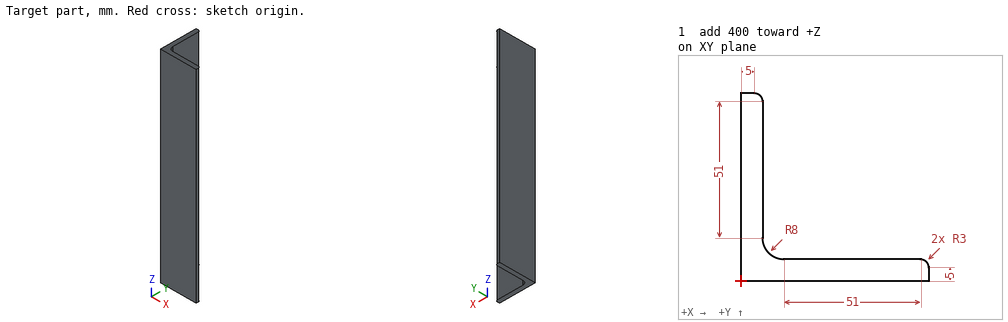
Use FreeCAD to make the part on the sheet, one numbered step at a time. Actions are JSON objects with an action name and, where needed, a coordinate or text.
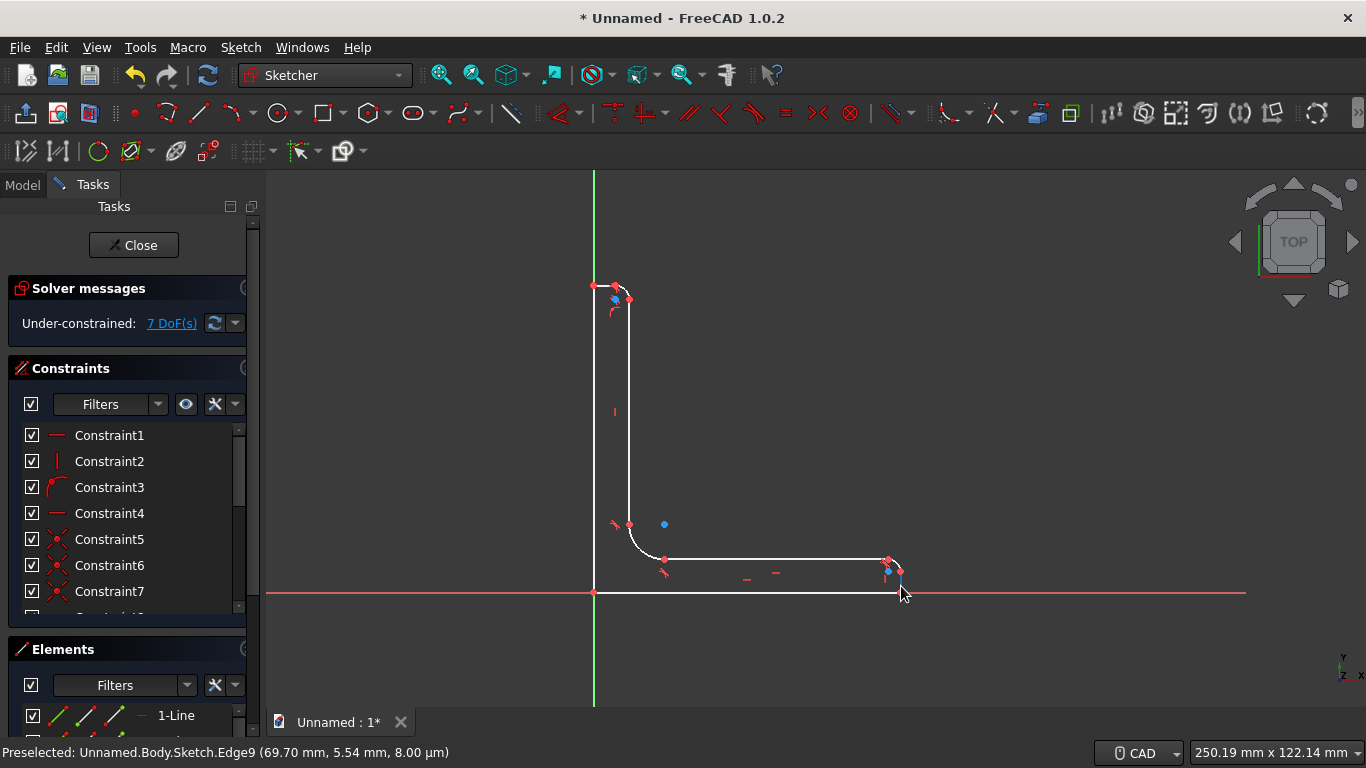
{"action": "scroll", "coordinate": [628, 293], "scroll_direction": "up", "scroll_amount": 4}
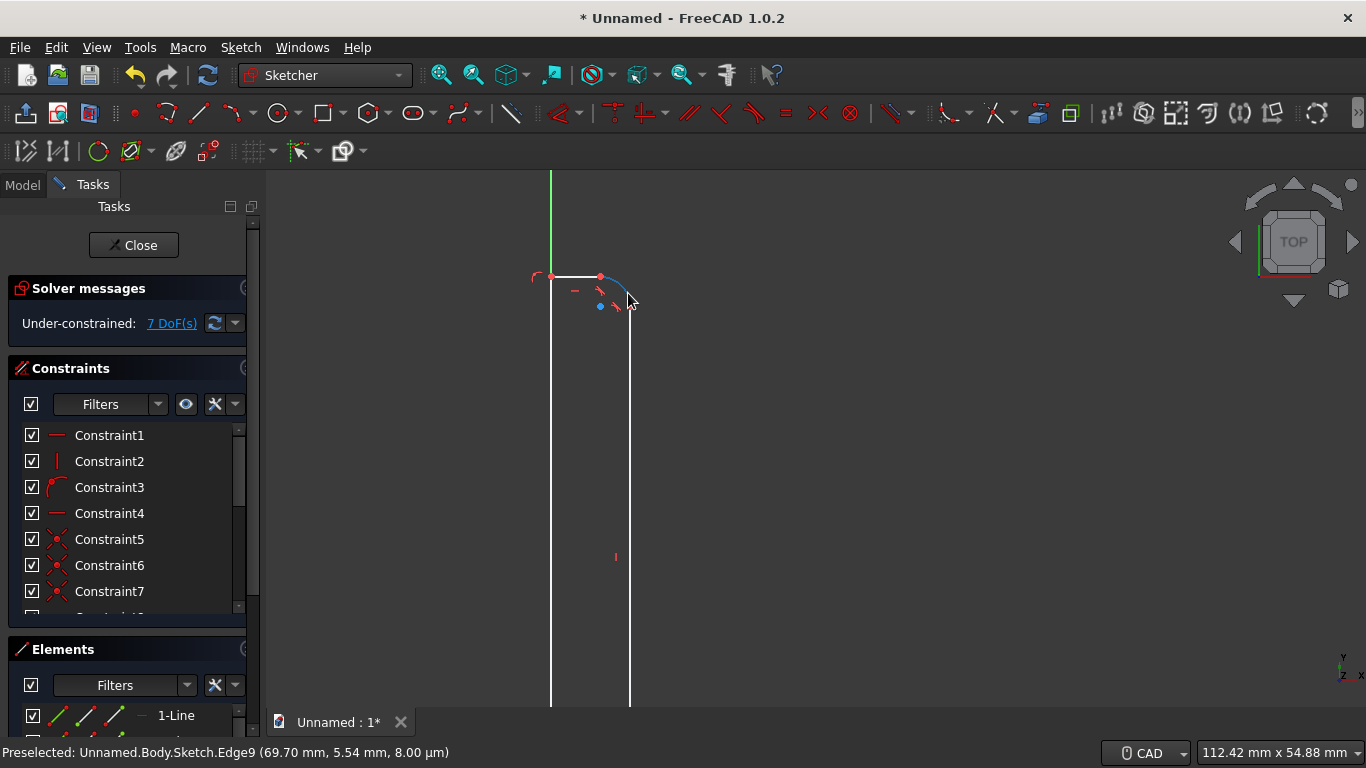
{"action": "left_click", "coordinate": [627, 293]}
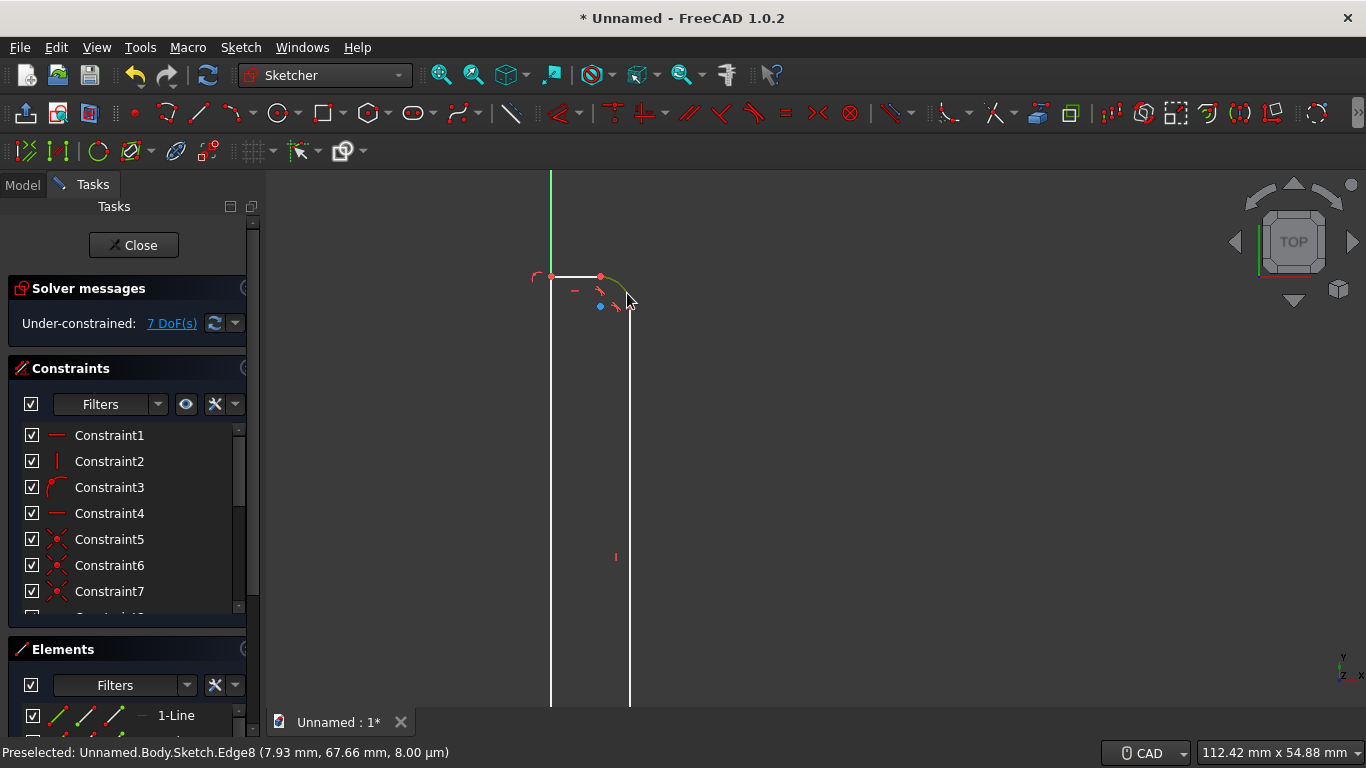
{"action": "scroll", "coordinate": [628, 293], "scroll_direction": "down", "scroll_amount": 4}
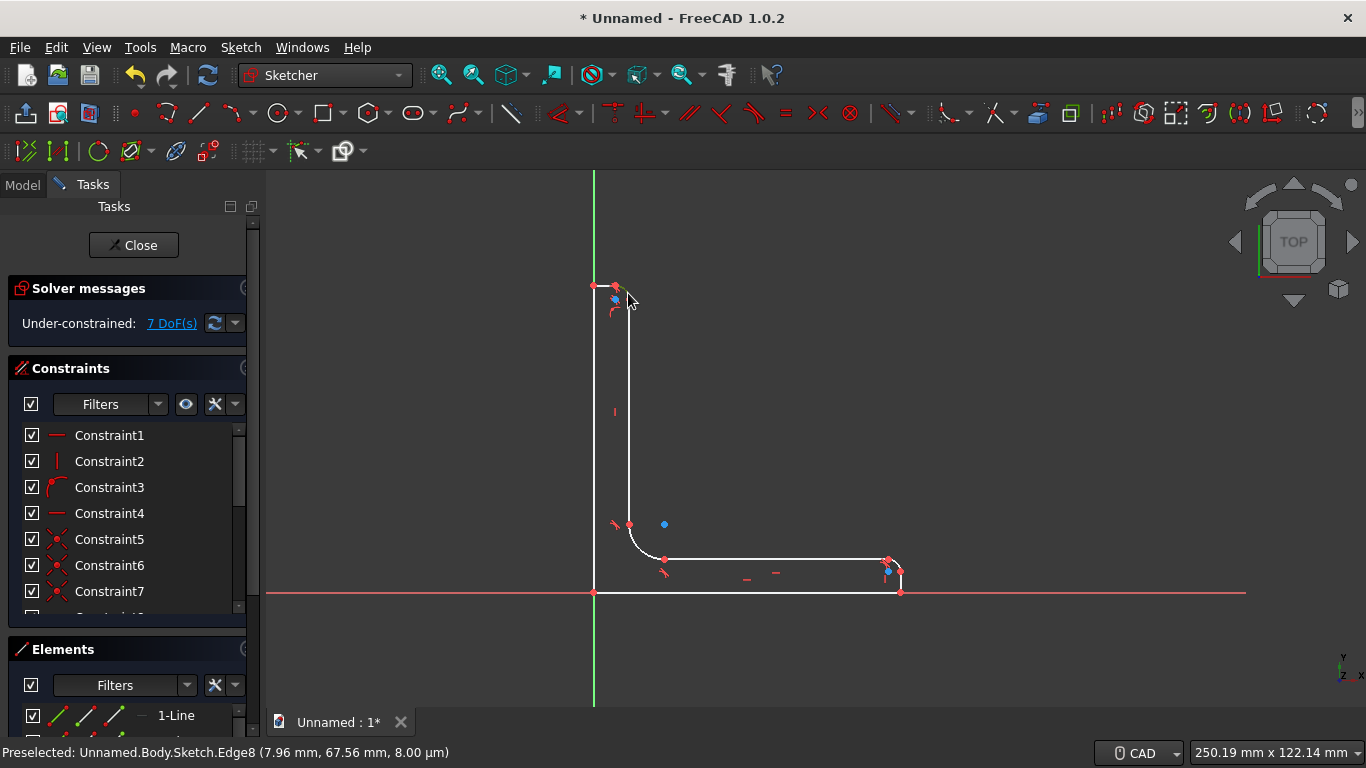
{"action": "scroll", "coordinate": [899, 566], "scroll_direction": "up", "scroll_amount": 5}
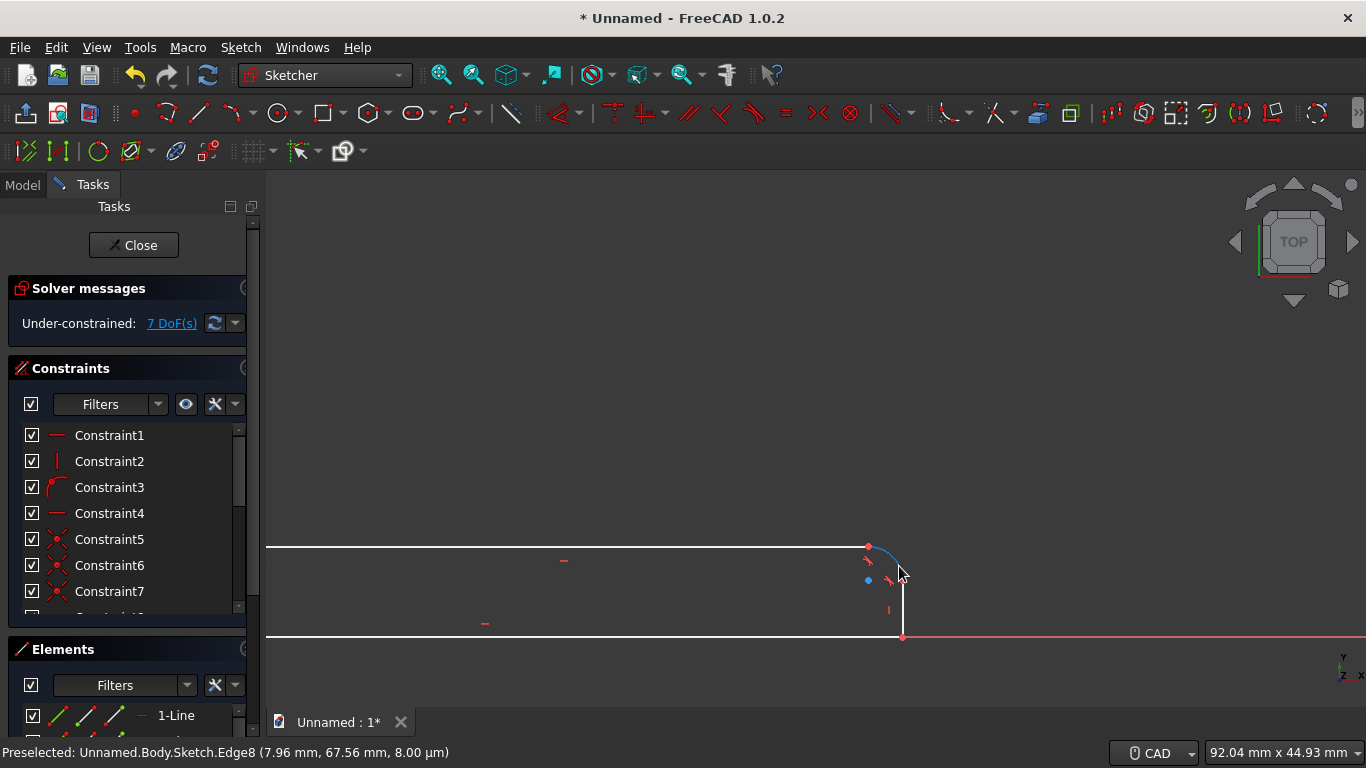
{"action": "left_click", "coordinate": [899, 565]}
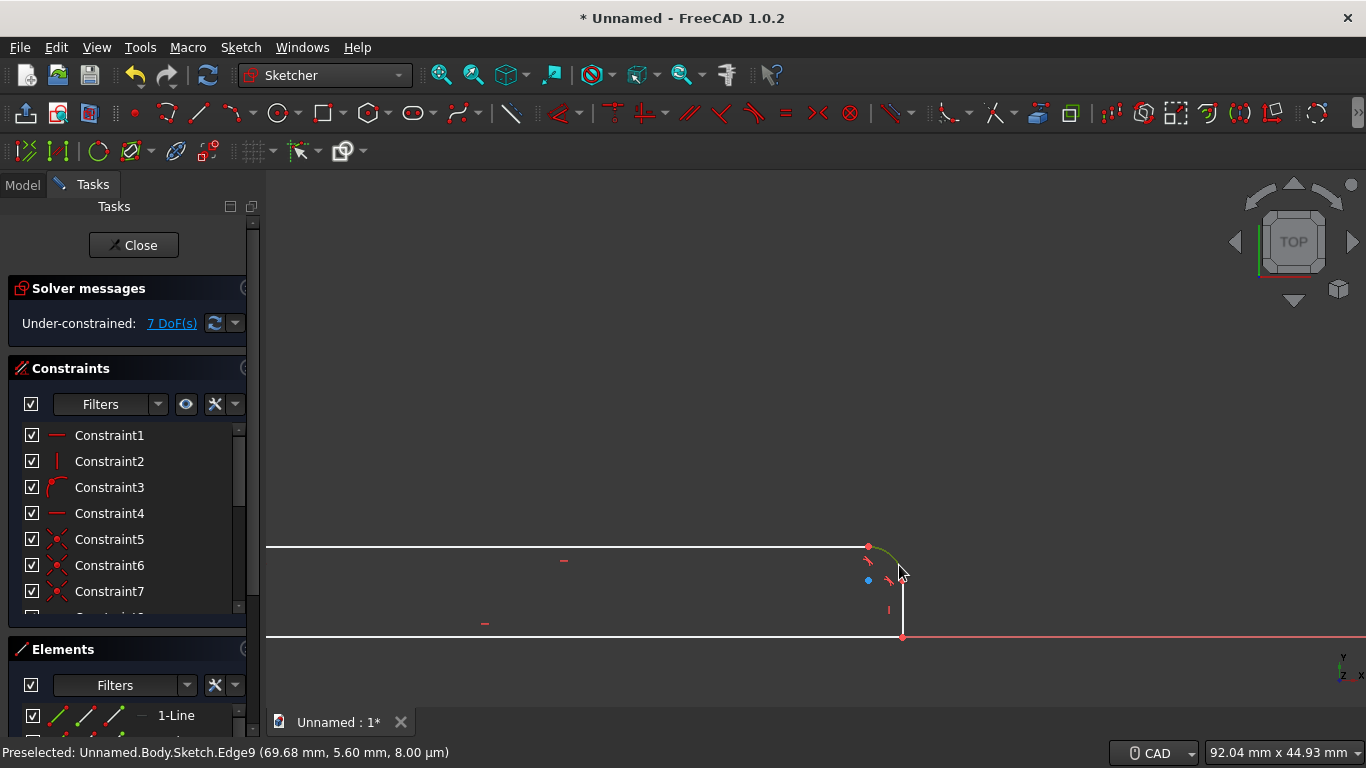
{"action": "left_click", "coordinate": [786, 114]}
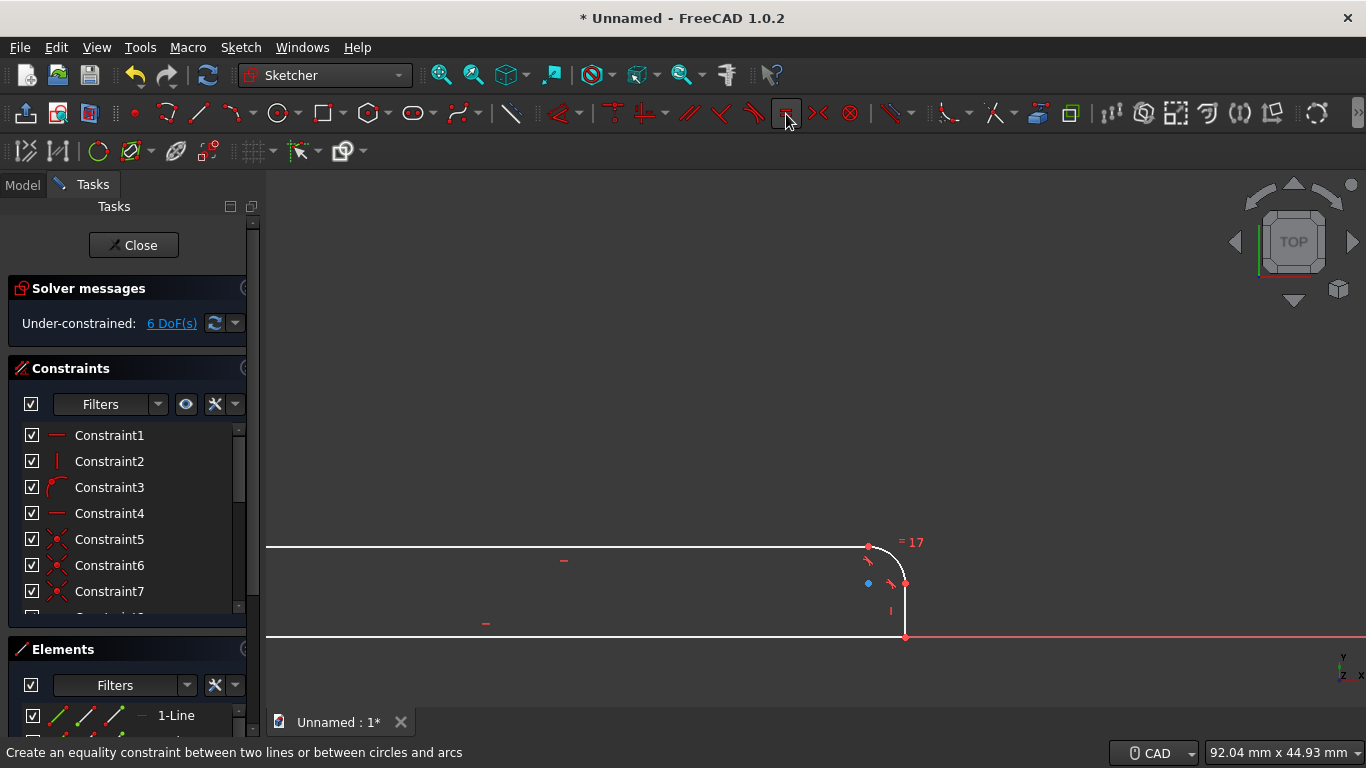
{"action": "left_click", "coordinate": [558, 114]}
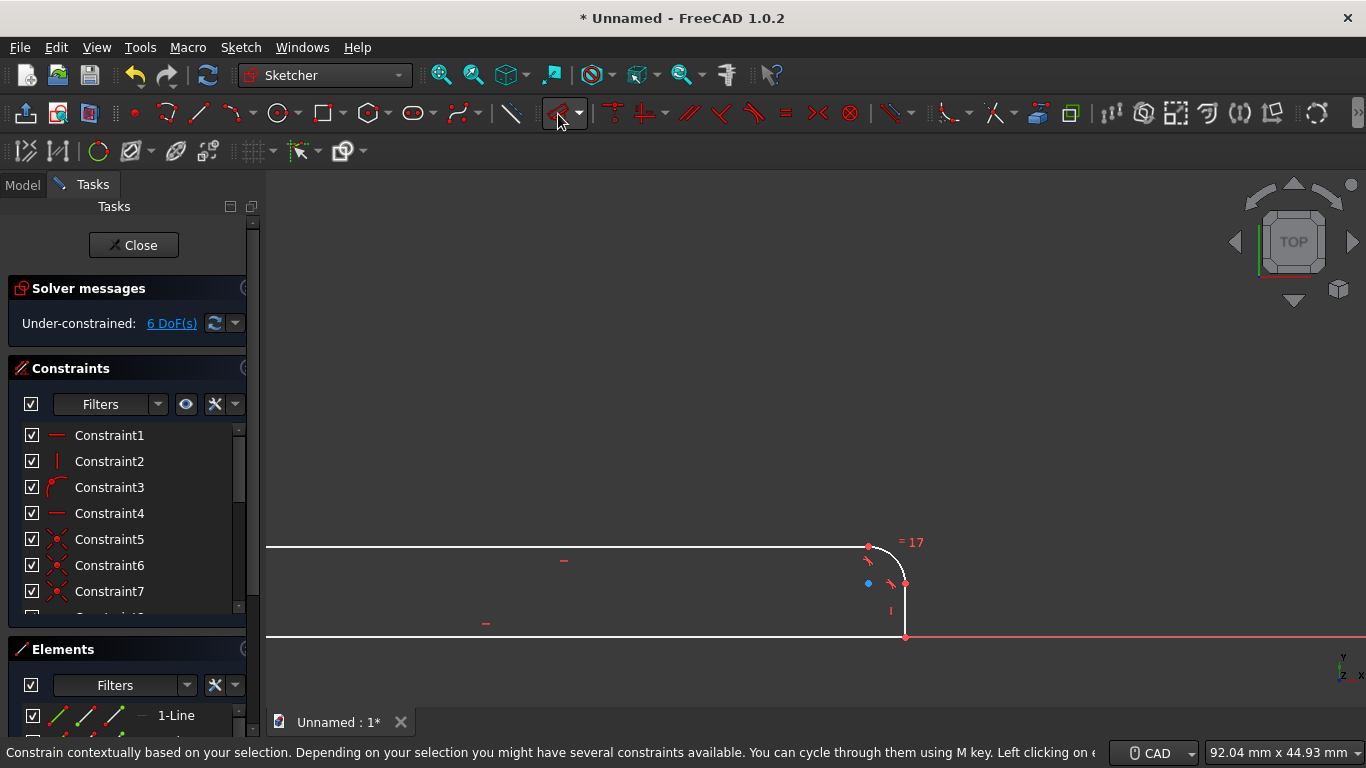
{"action": "scroll", "coordinate": [899, 566], "scroll_direction": "down", "scroll_amount": 5}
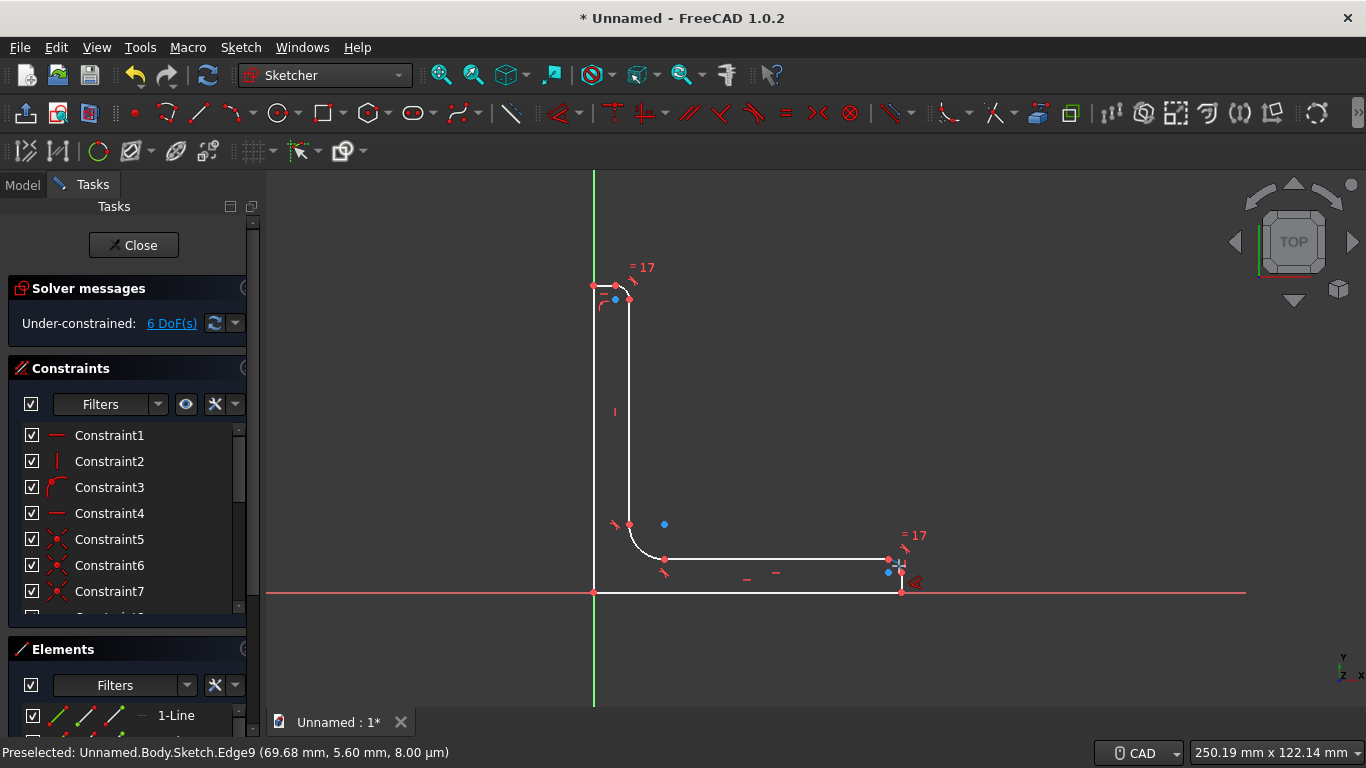
{"action": "left_click", "coordinate": [633, 540]}
{"action": "left_click", "coordinate": [626, 580]}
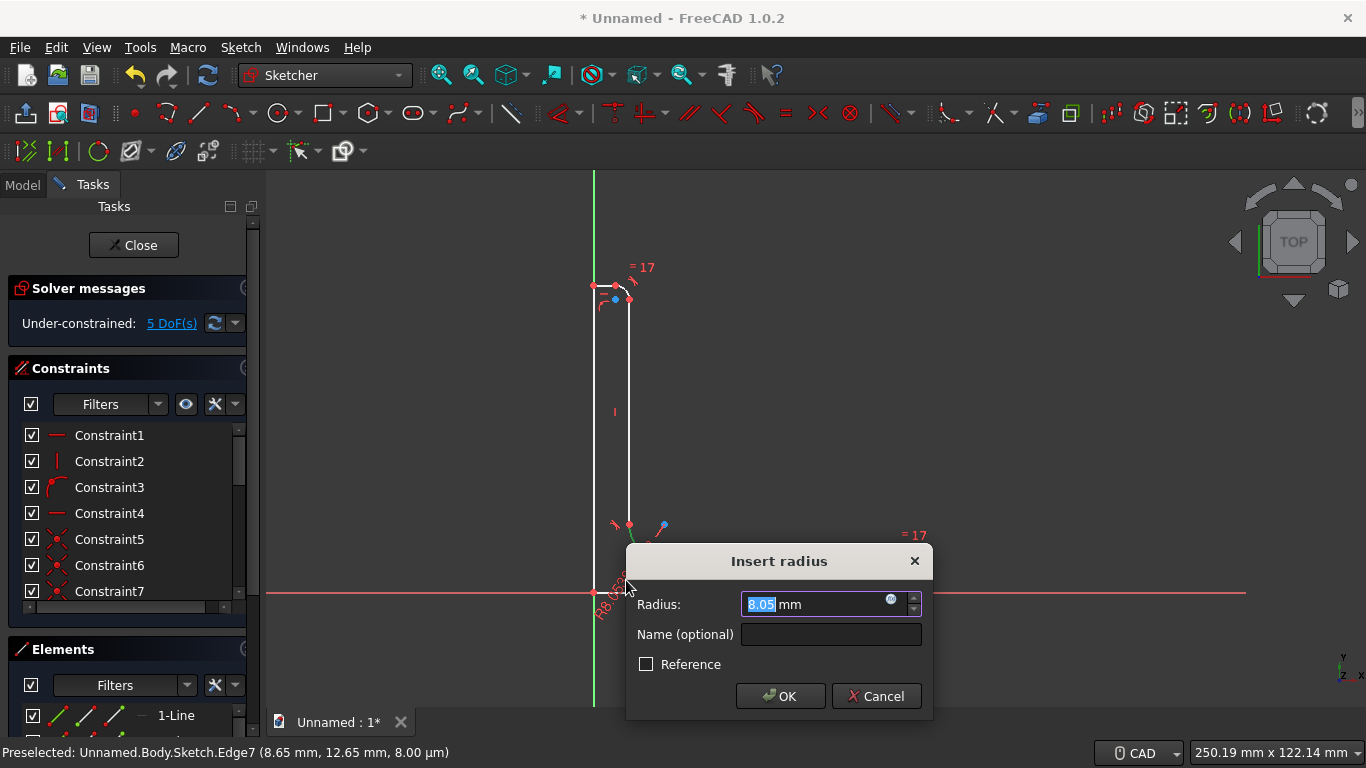
{"action": "type", "text": "8"}
{"action": "key", "text": "Return"}